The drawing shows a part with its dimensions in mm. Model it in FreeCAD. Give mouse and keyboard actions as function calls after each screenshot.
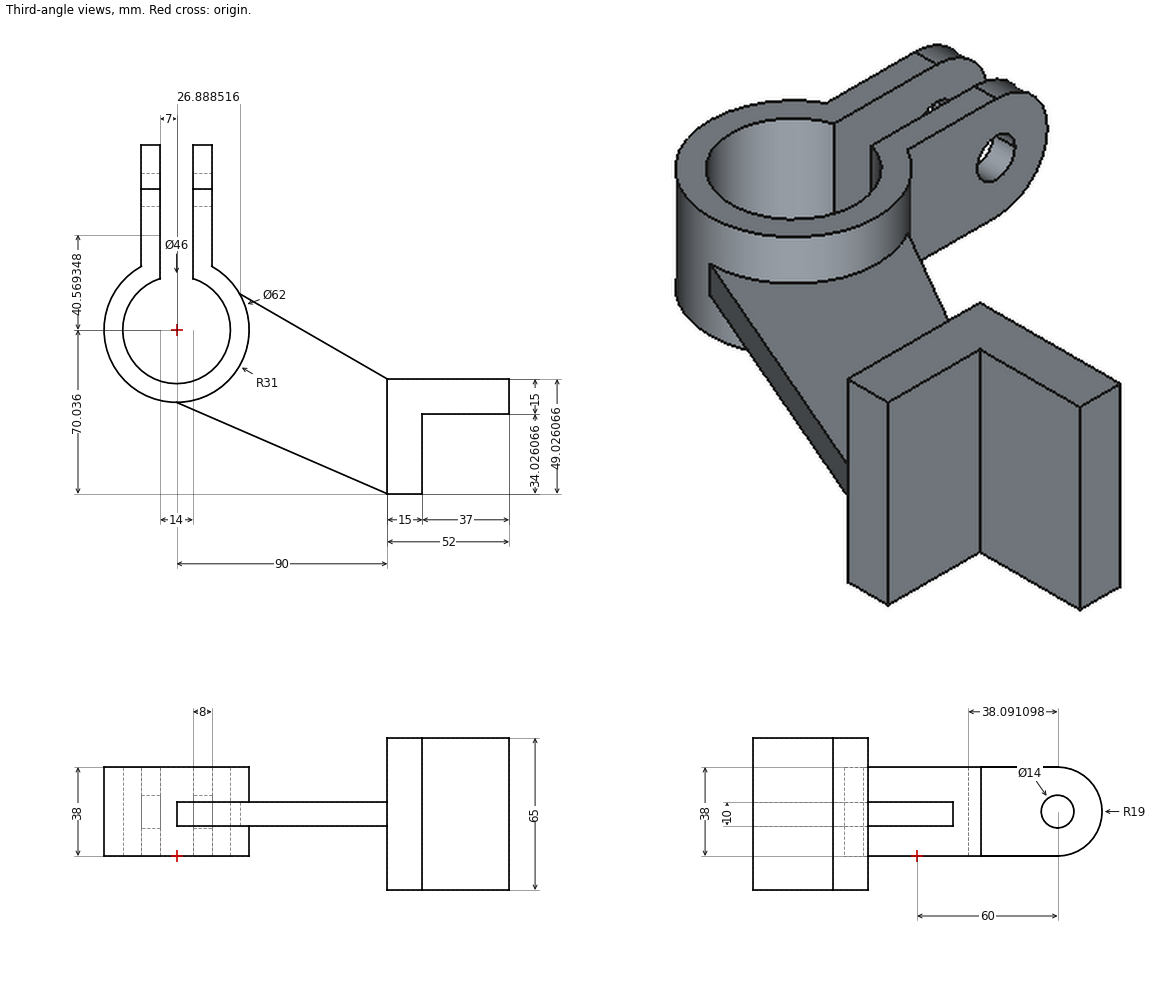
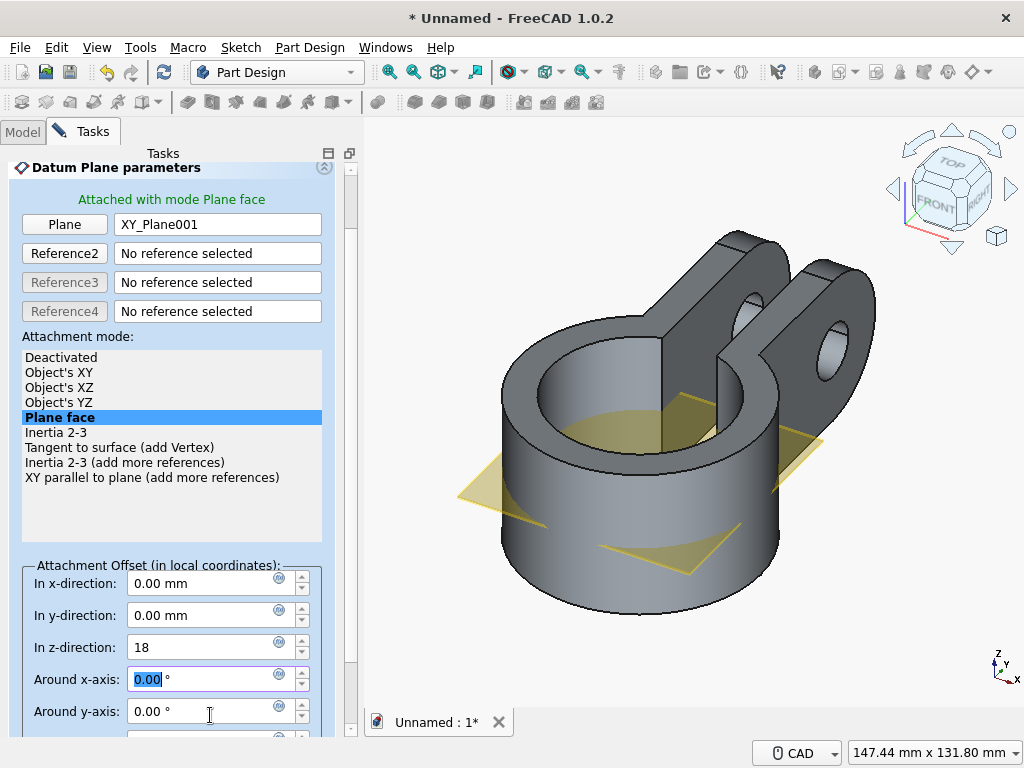
scroll(351, 450, up, 2)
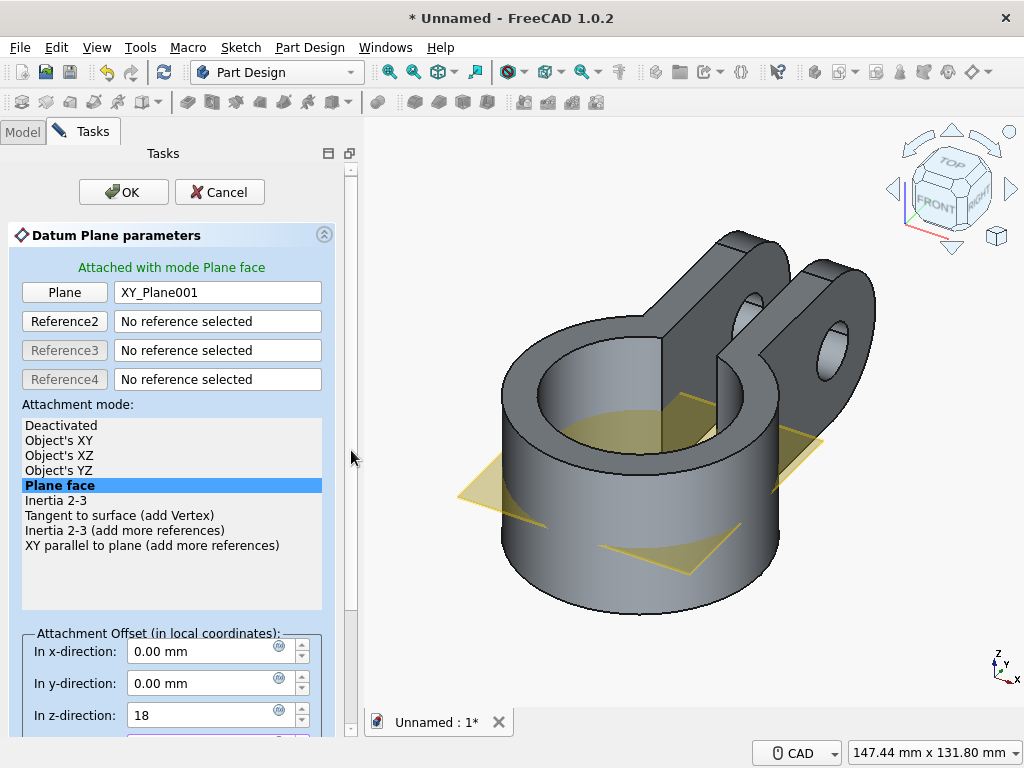
click(124, 192)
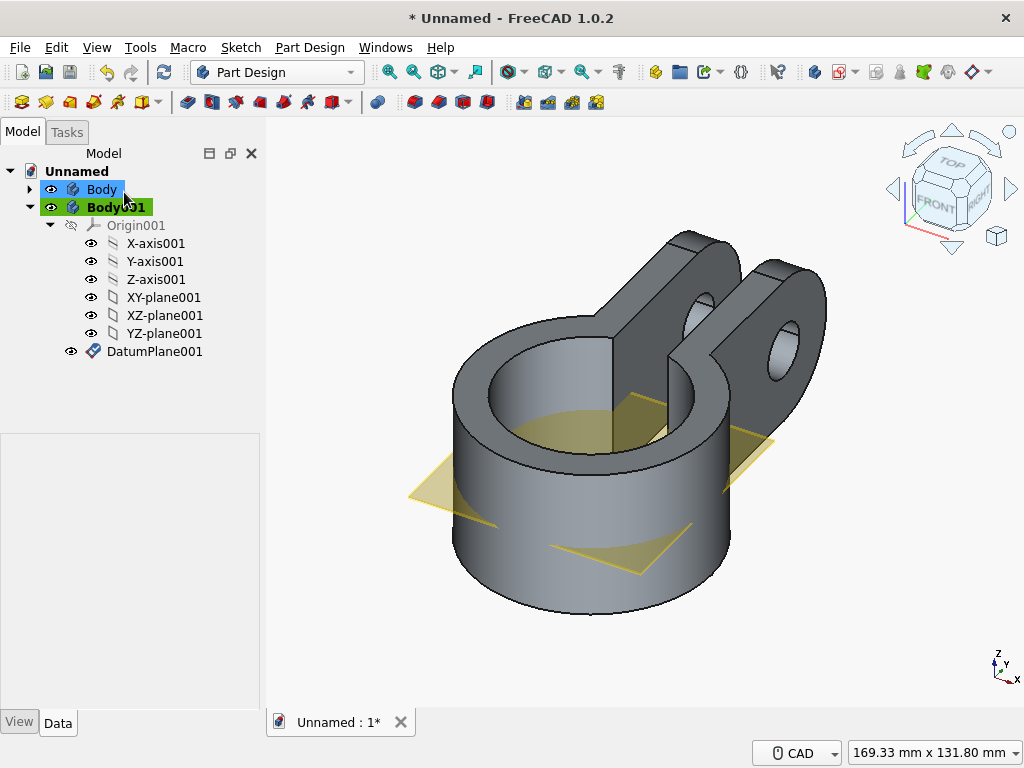
click(116, 351)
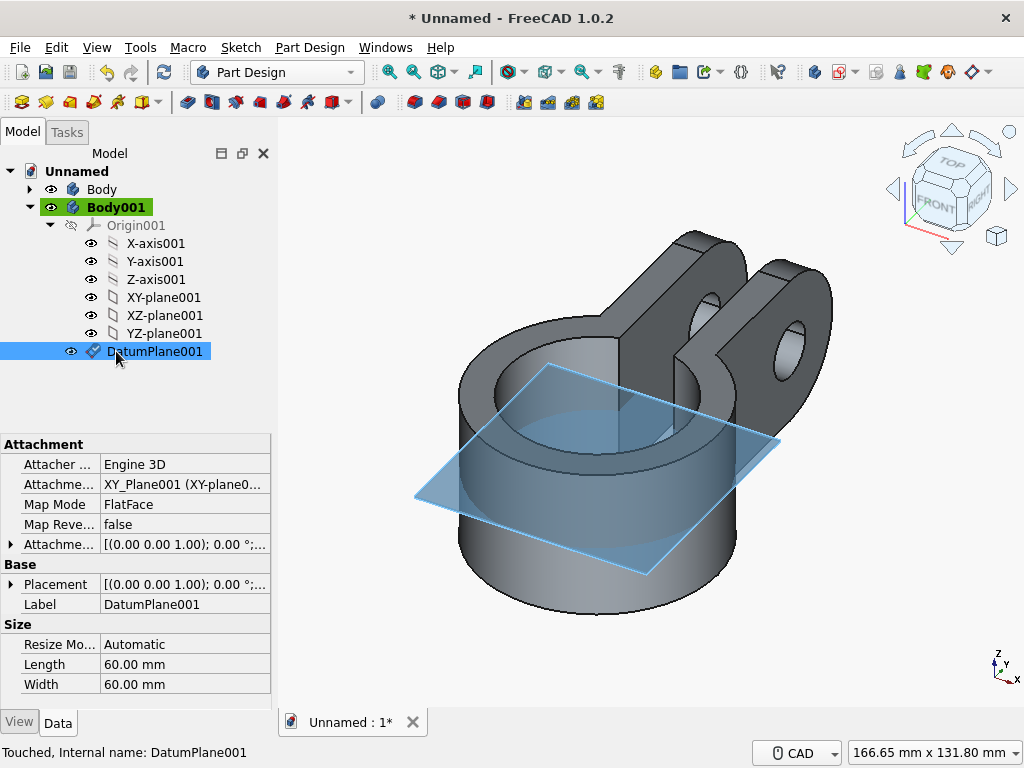
click(840, 72)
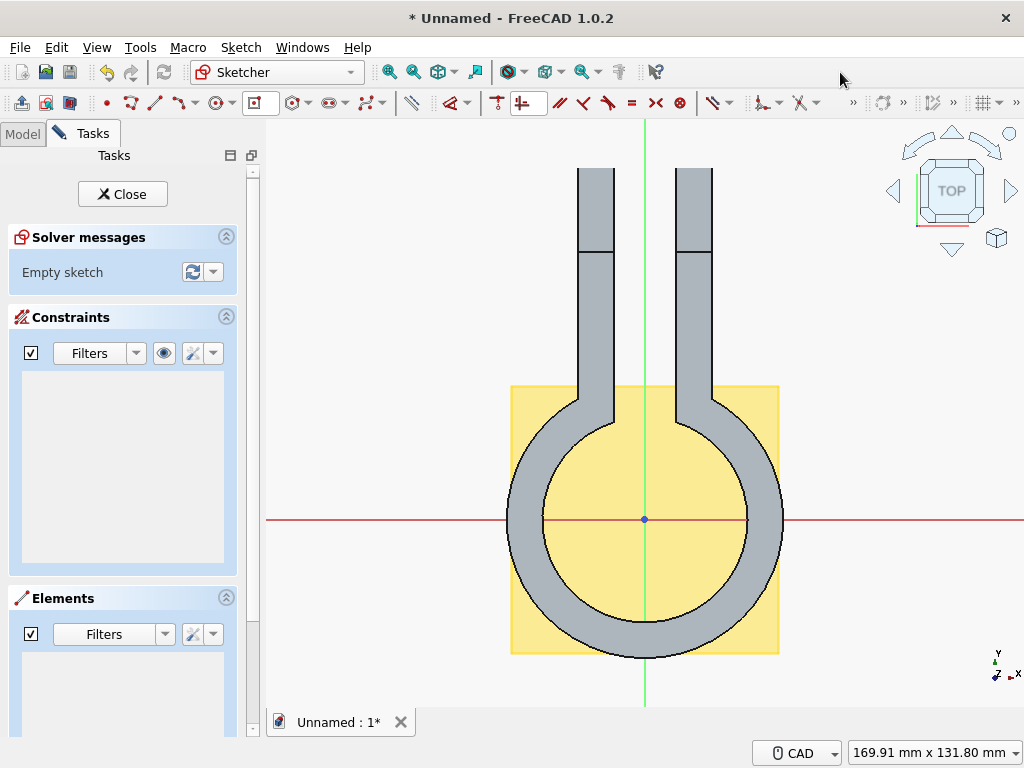
scroll(576, 413, down, 5)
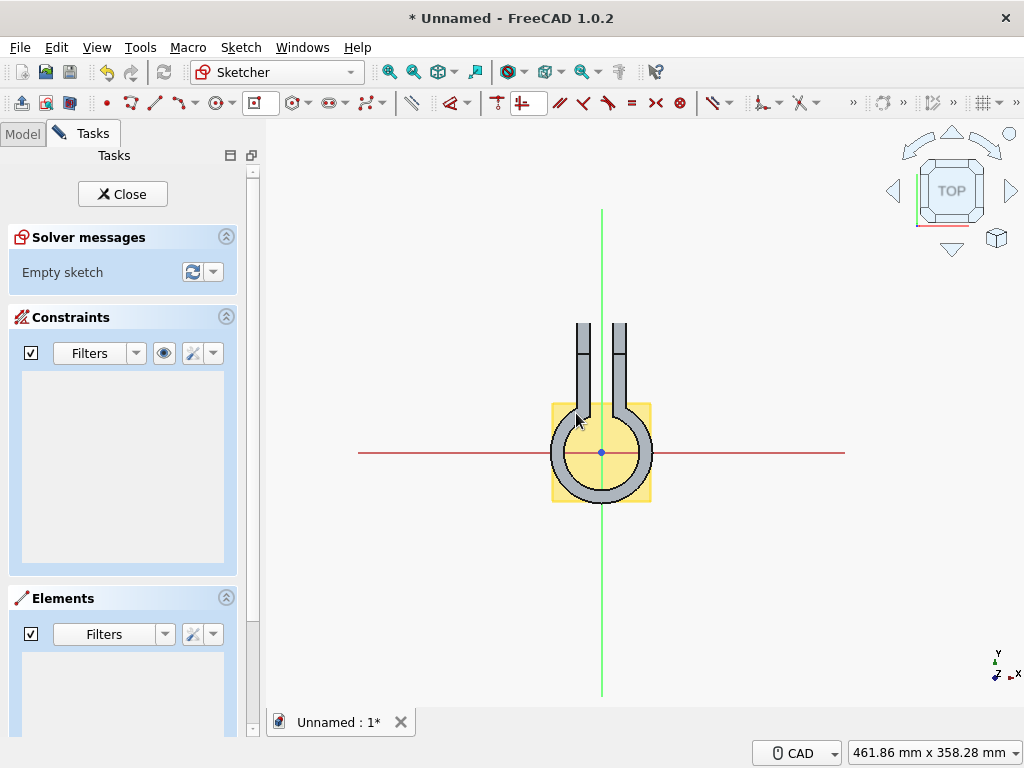
scroll(847, 556, up, 8)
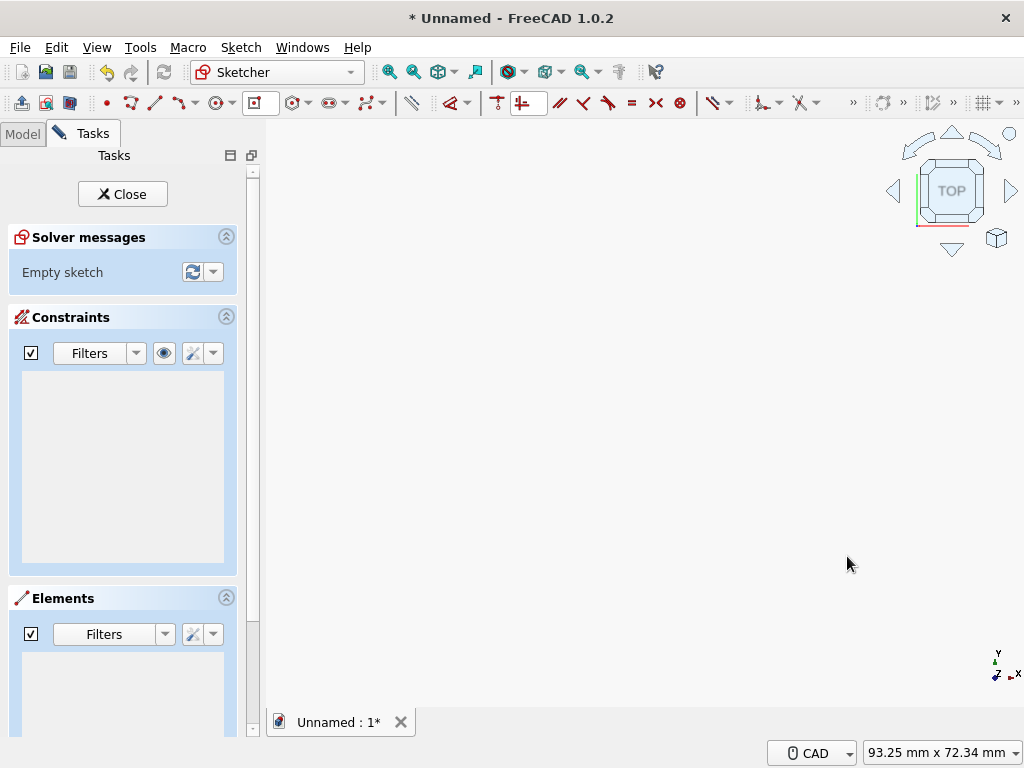
click(132, 104)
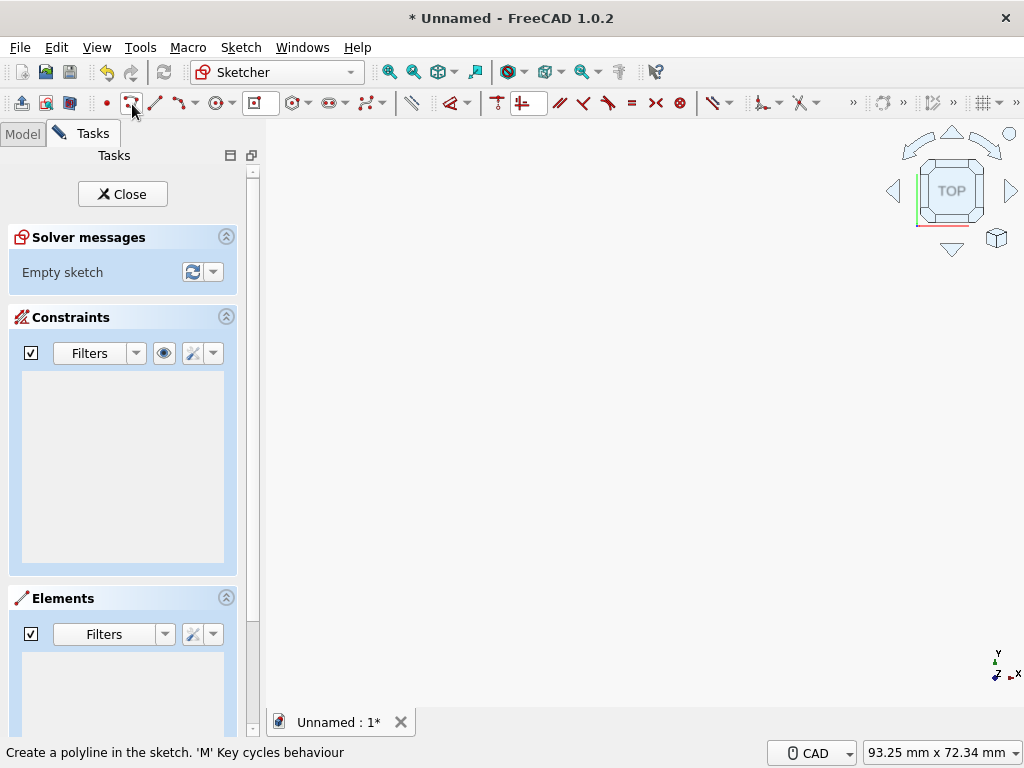
click(360, 212)
click(360, 610)
click(482, 610)
click(482, 334)
click(783, 334)
click(783, 212)
click(360, 213)
key(Escape)
key(Escape)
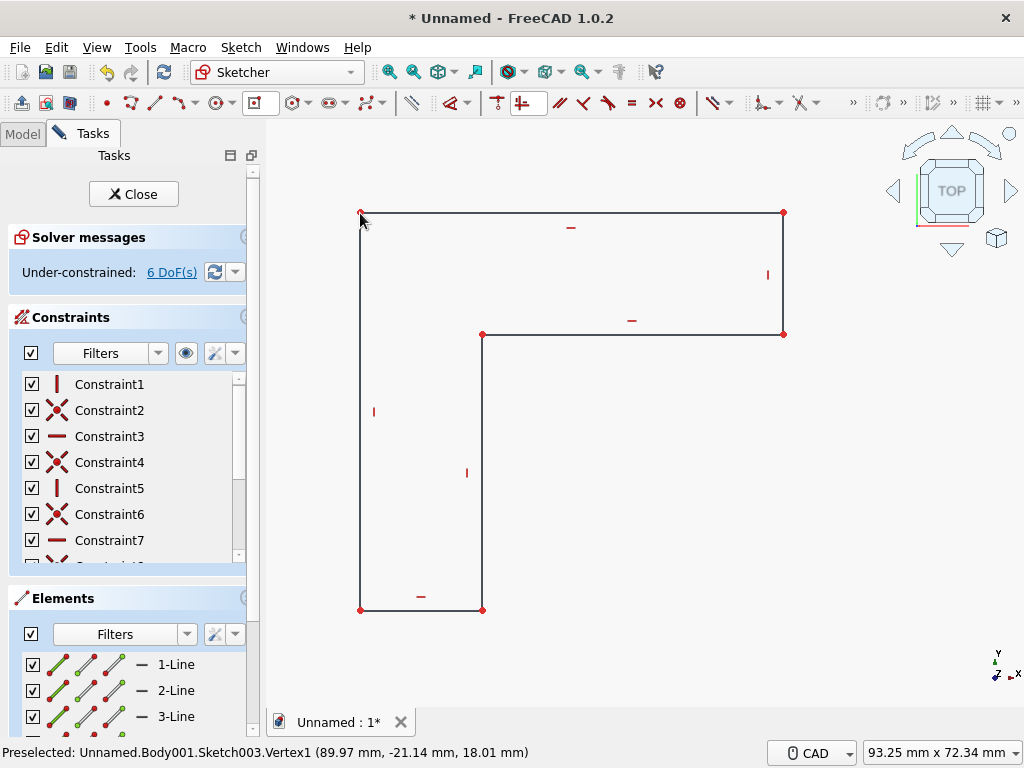
click(450, 104)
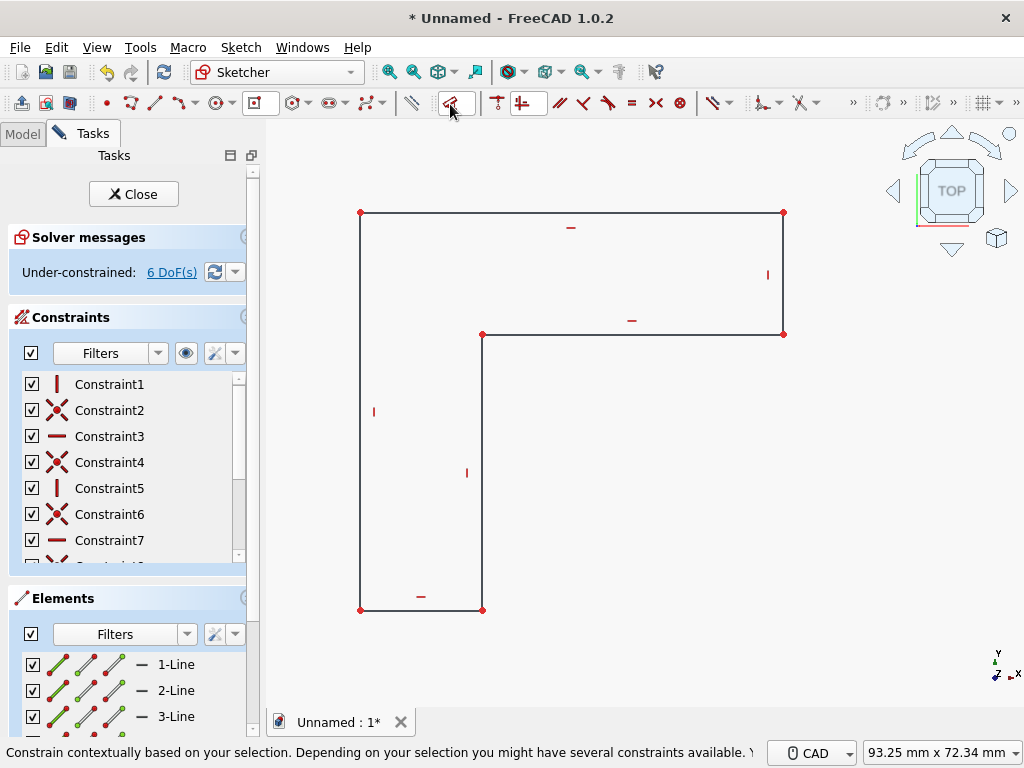
click(397, 611)
click(421, 645)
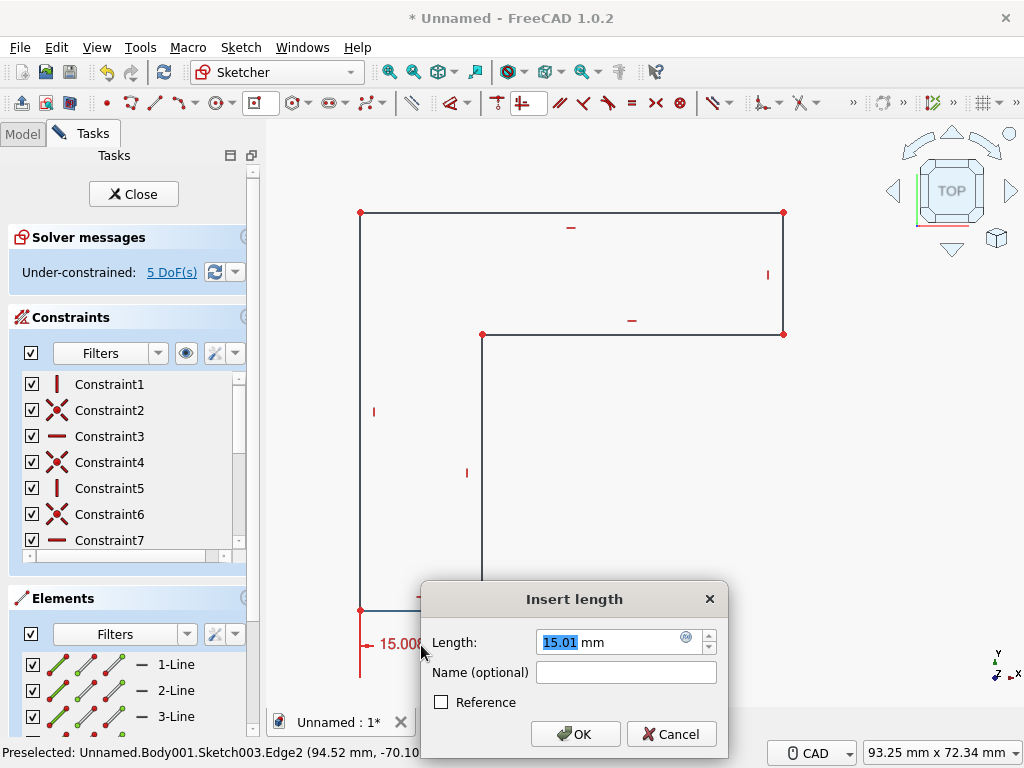
text(15)
key(Return)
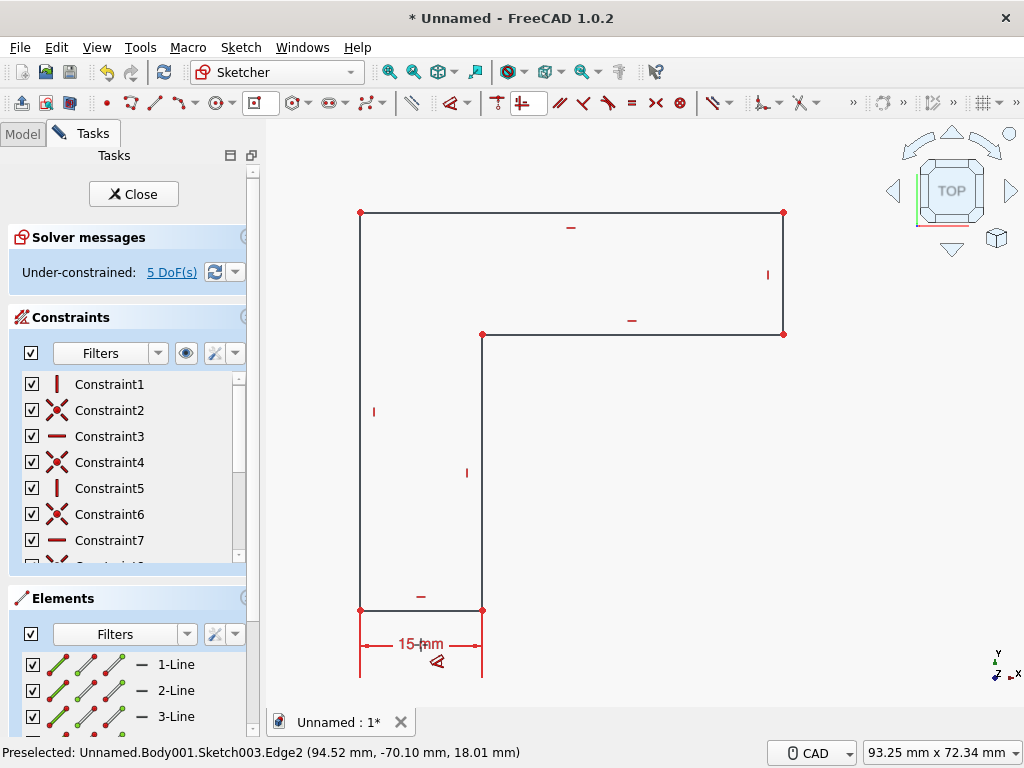
click(572, 335)
click(632, 301)